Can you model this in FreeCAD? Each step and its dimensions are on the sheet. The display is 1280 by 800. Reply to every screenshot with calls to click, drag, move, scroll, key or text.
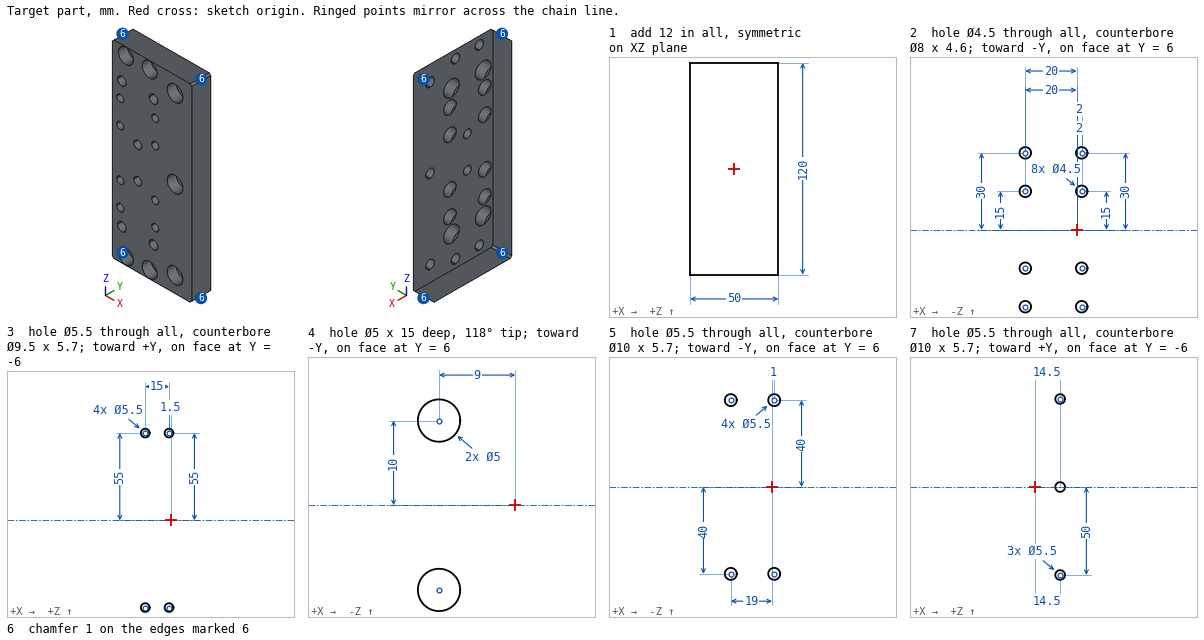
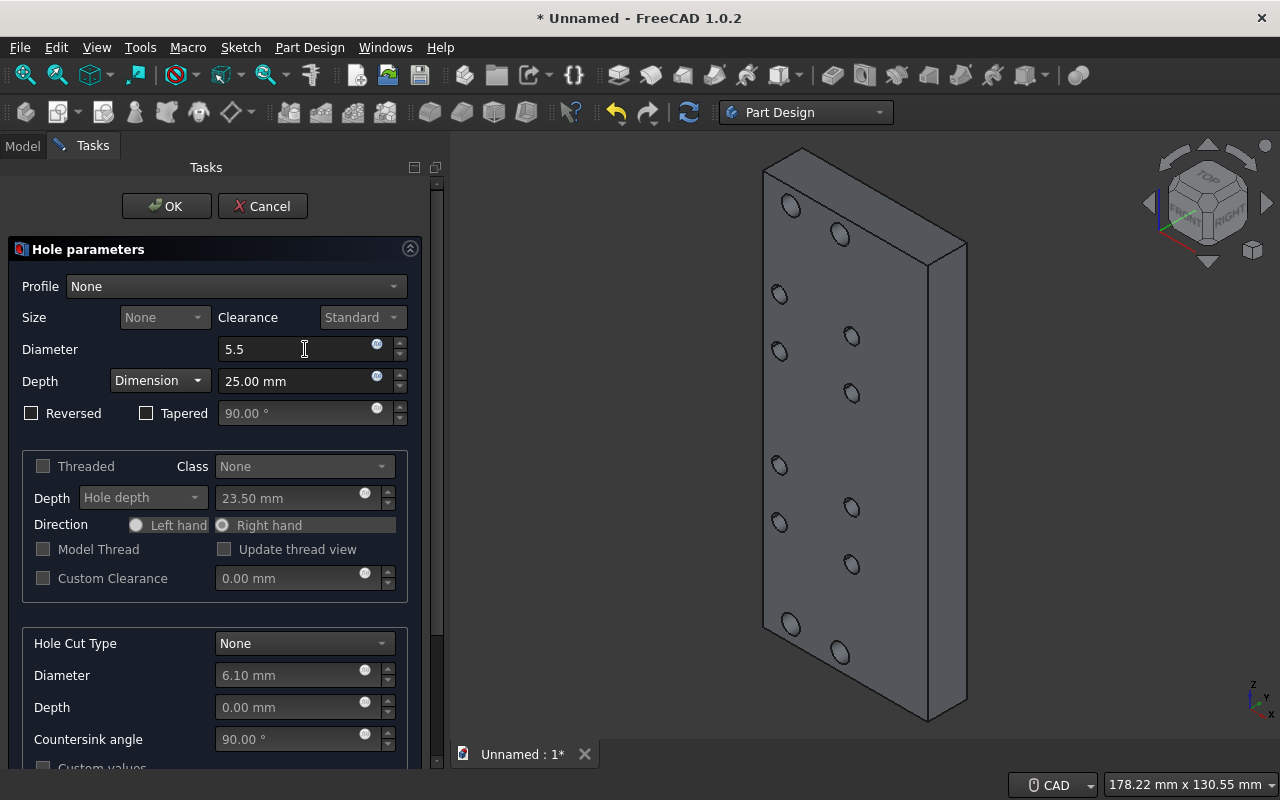
click(161, 380)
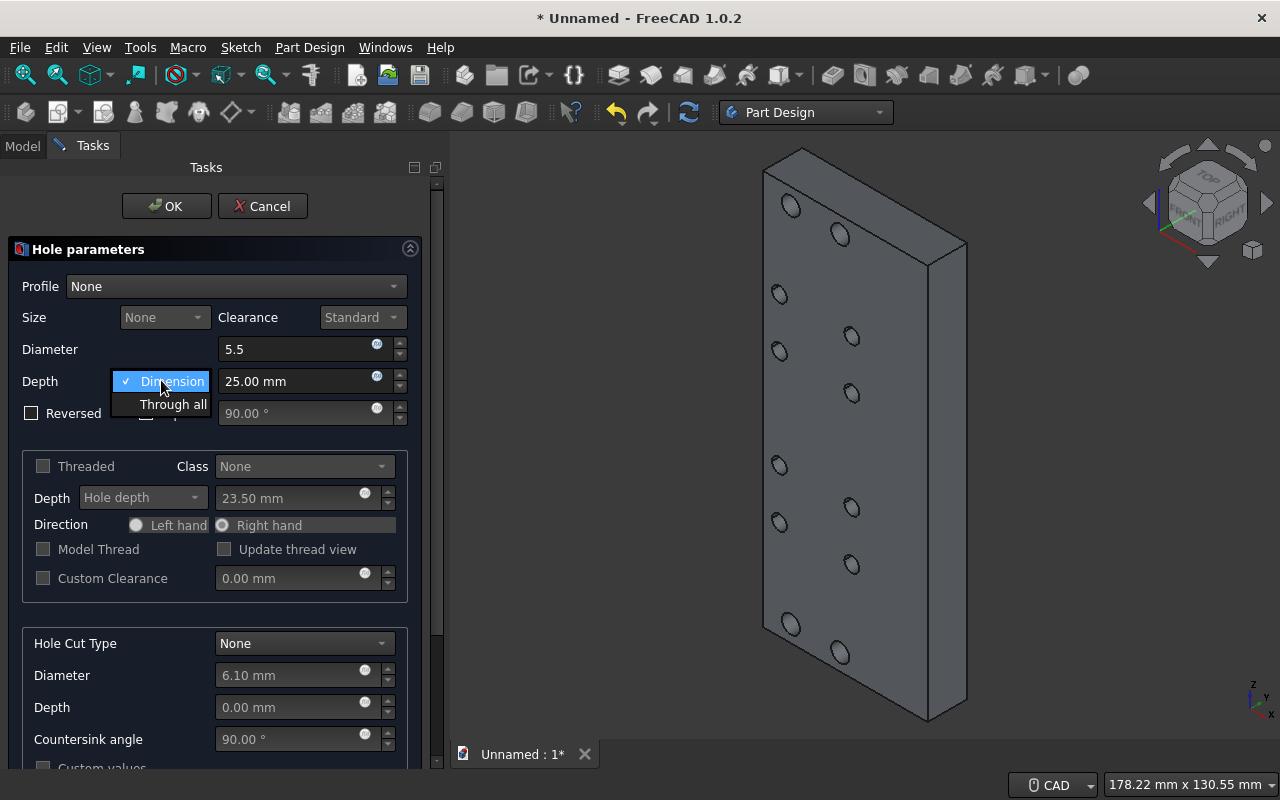
click(160, 404)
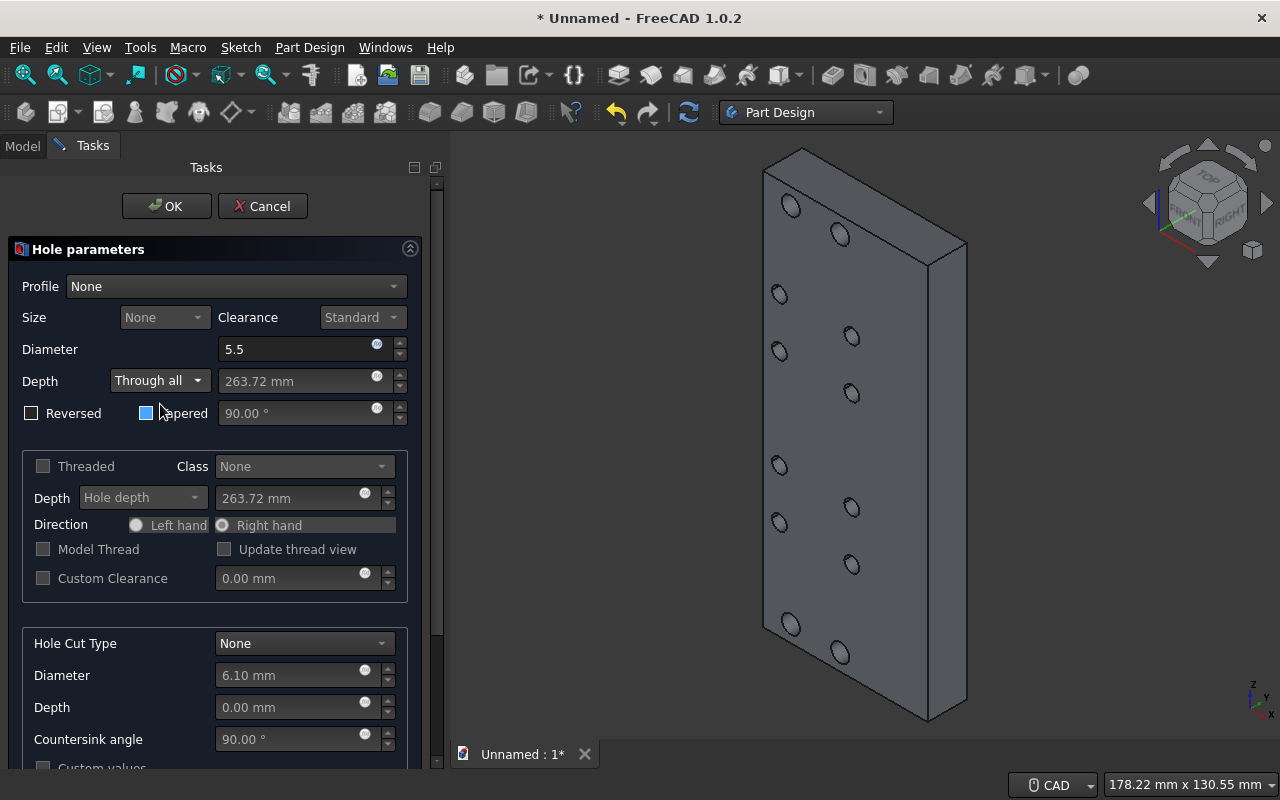
click(306, 644)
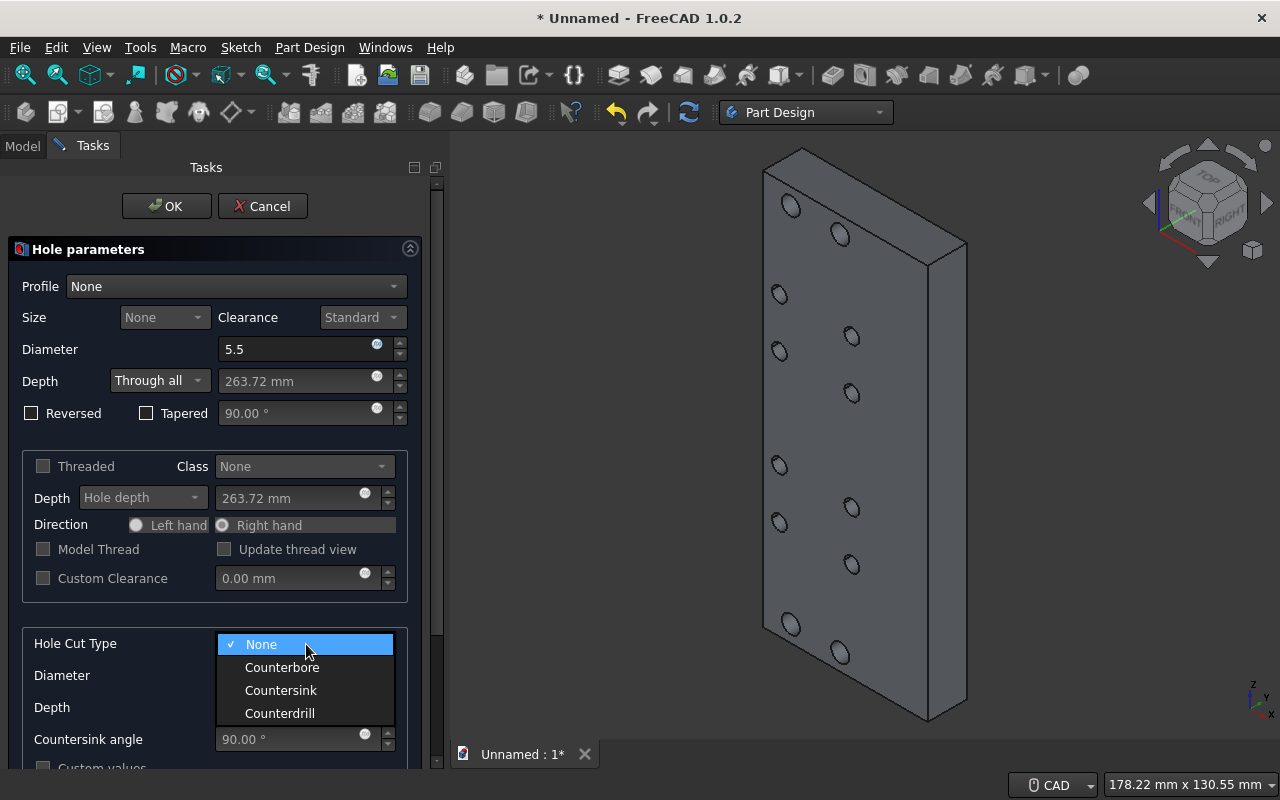
click(304, 668)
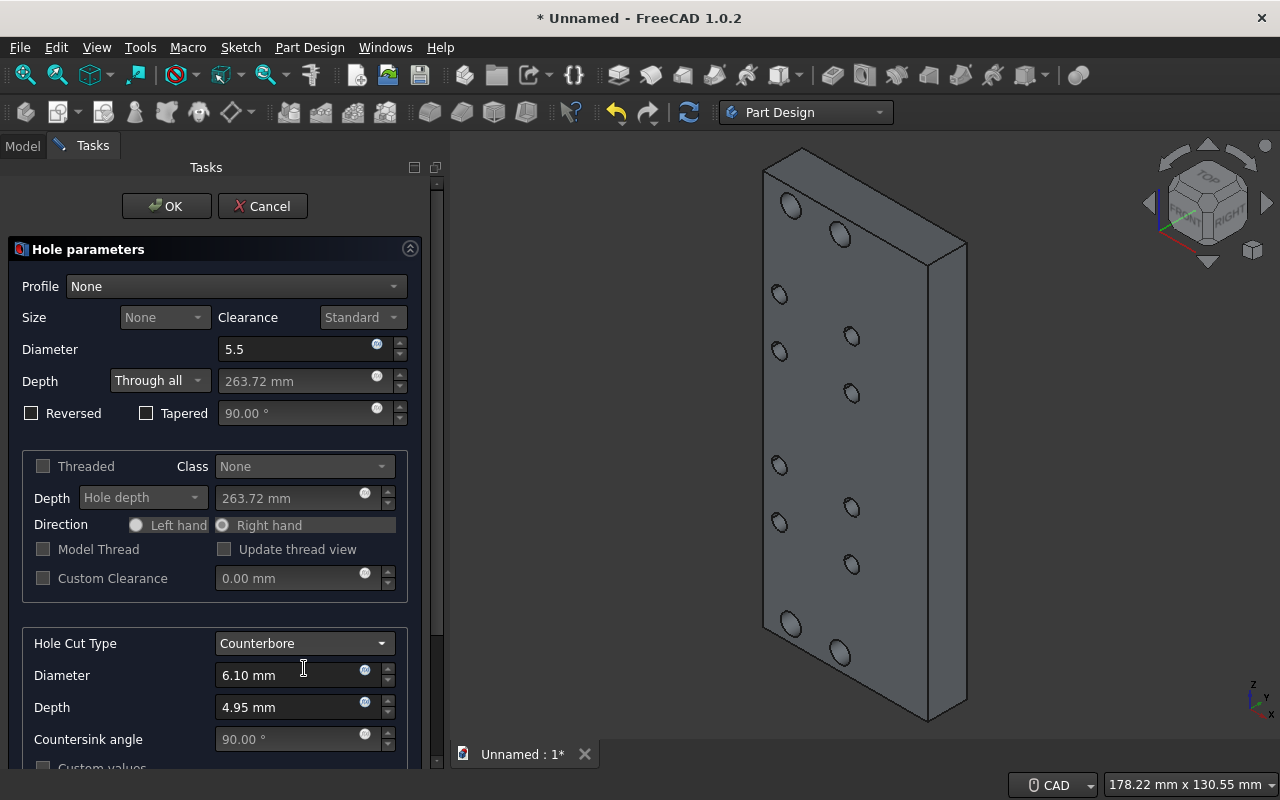
triple_click(298, 675)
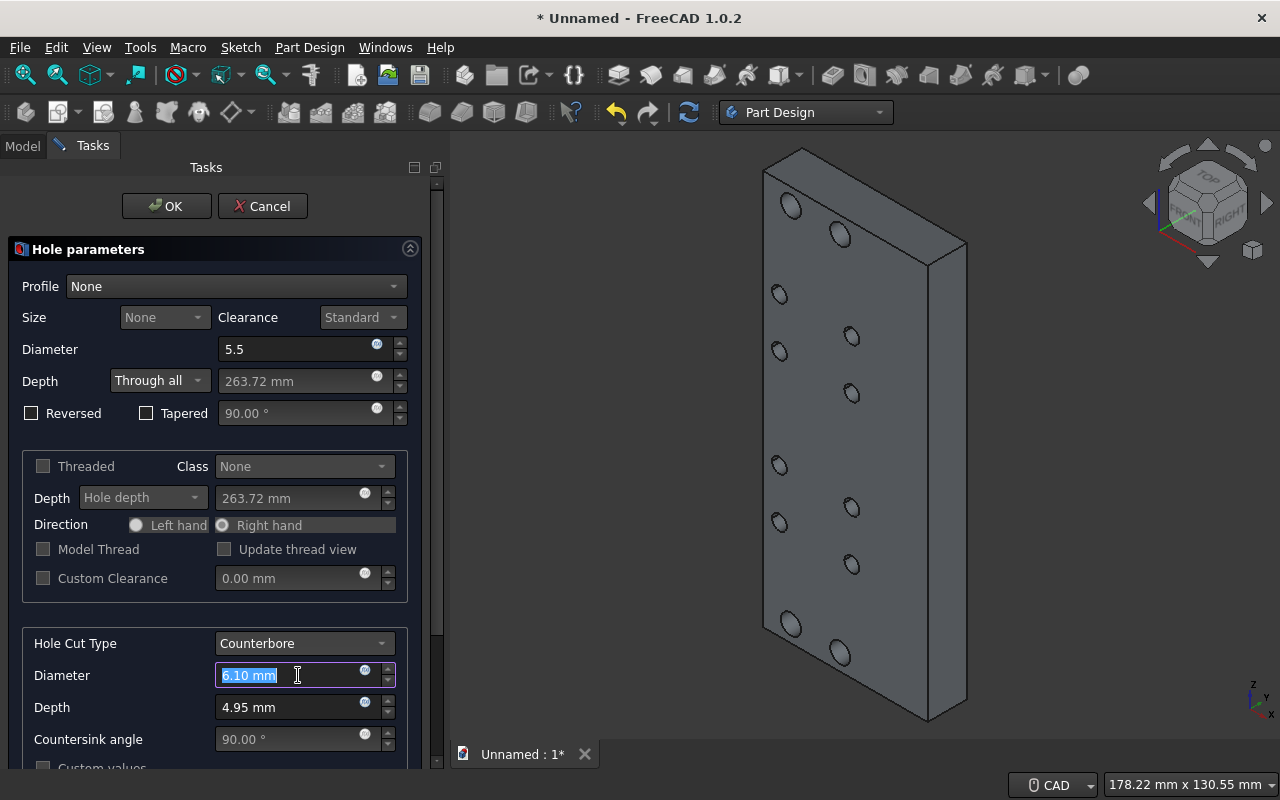
text(9.5)
key(Tab)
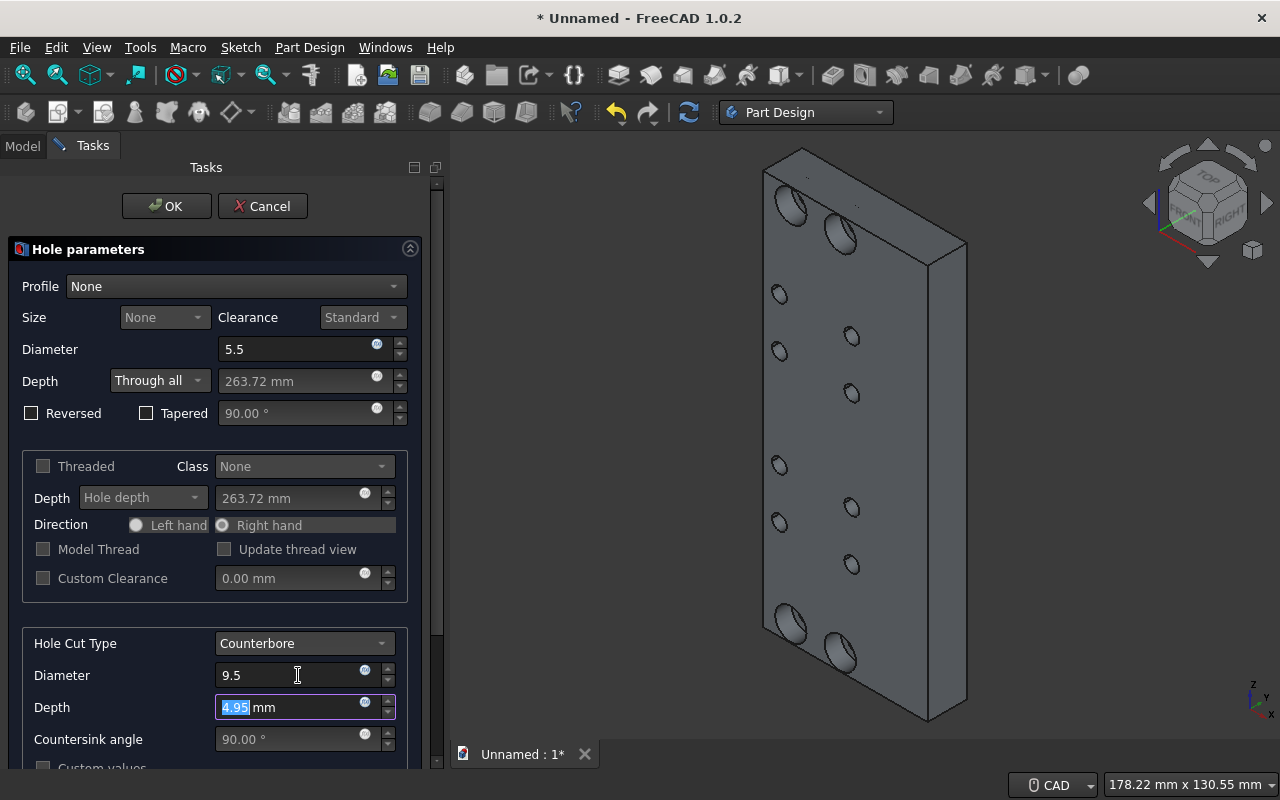
text(5.7)
key(Tab)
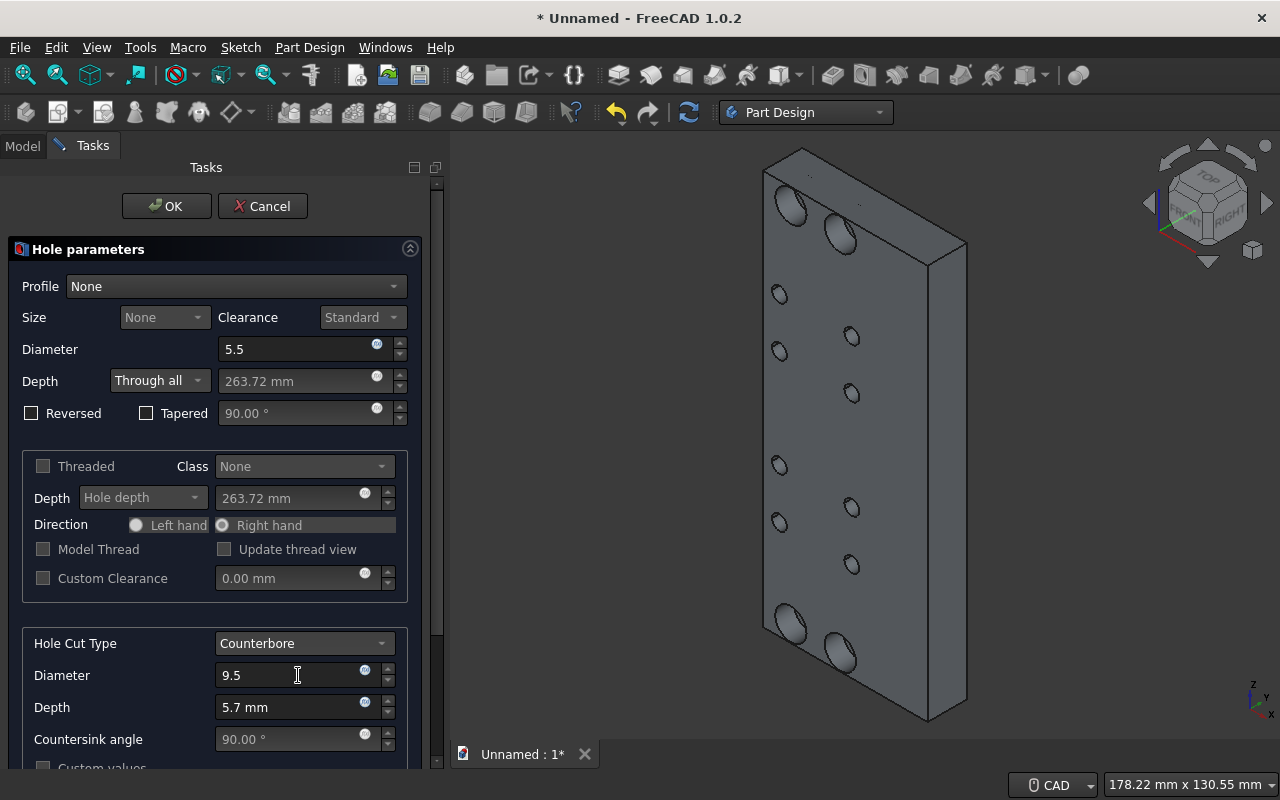
click(167, 206)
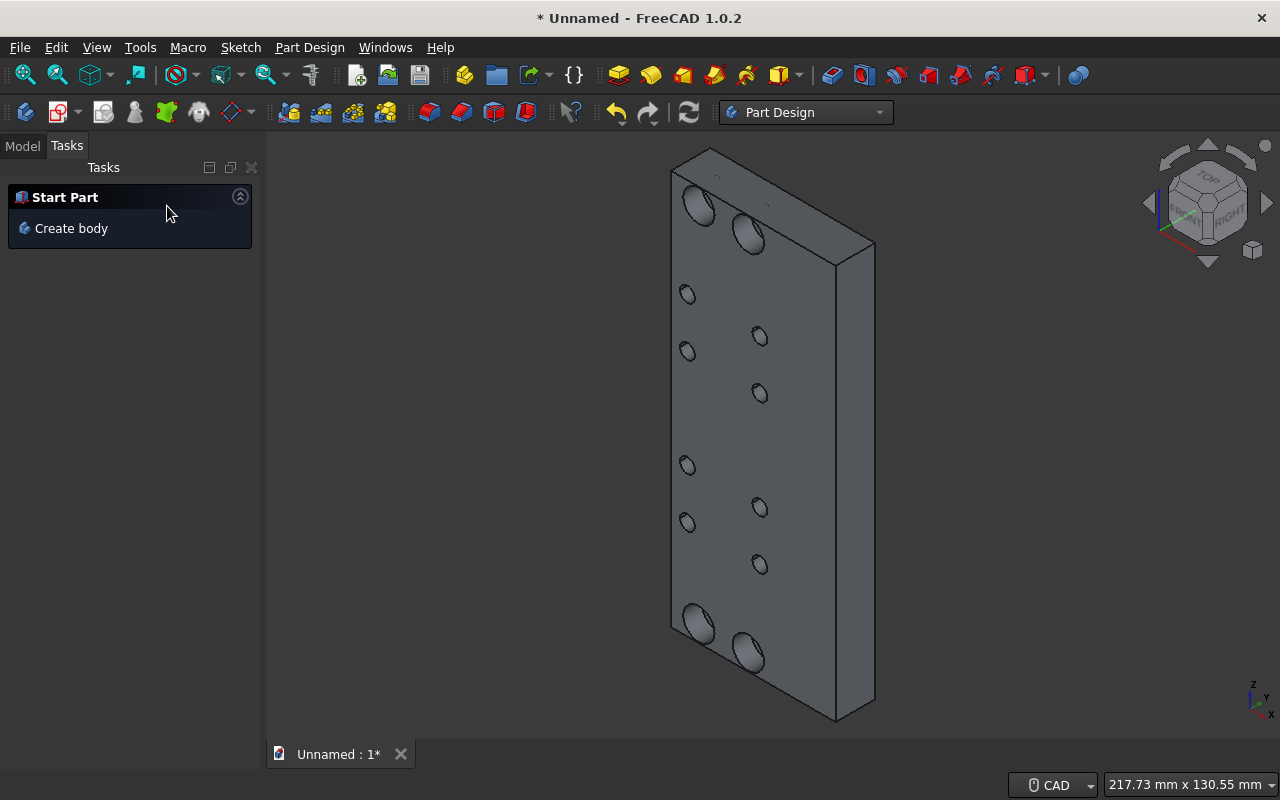
key(4)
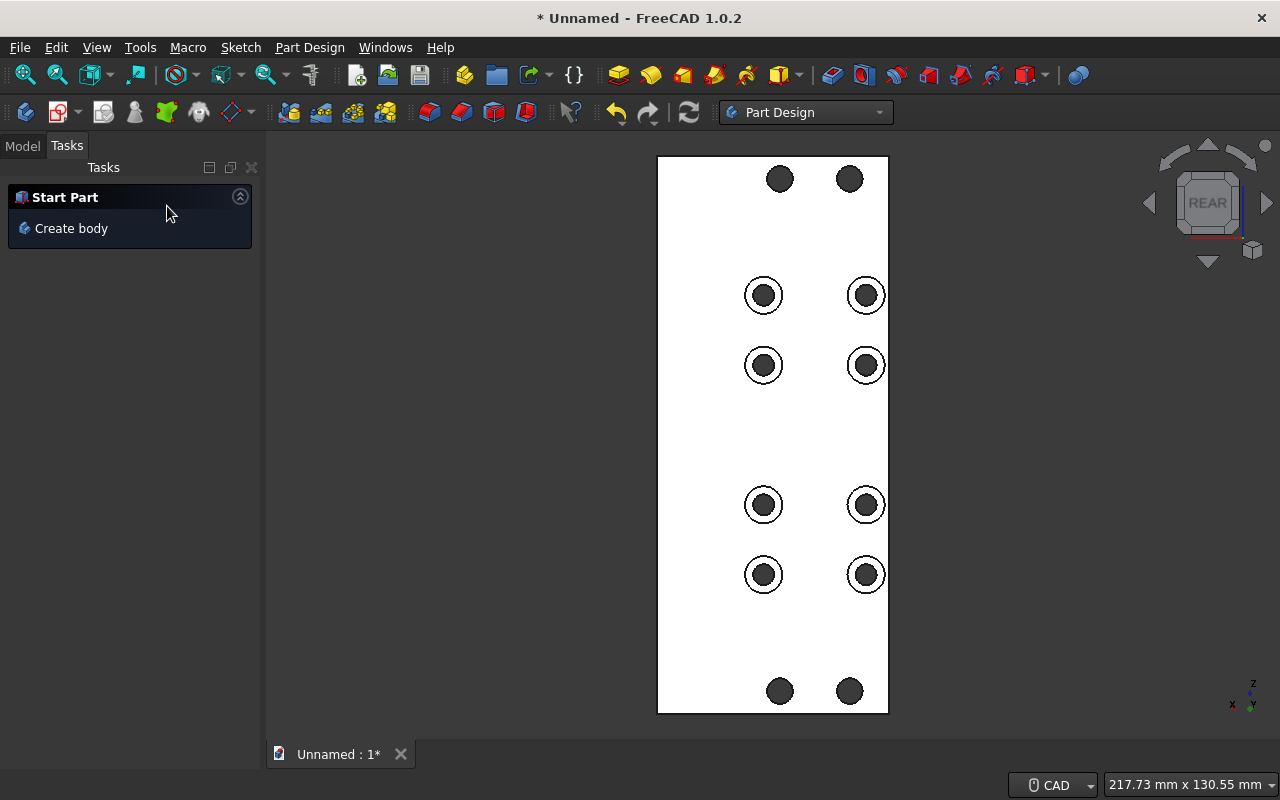
click(806, 434)